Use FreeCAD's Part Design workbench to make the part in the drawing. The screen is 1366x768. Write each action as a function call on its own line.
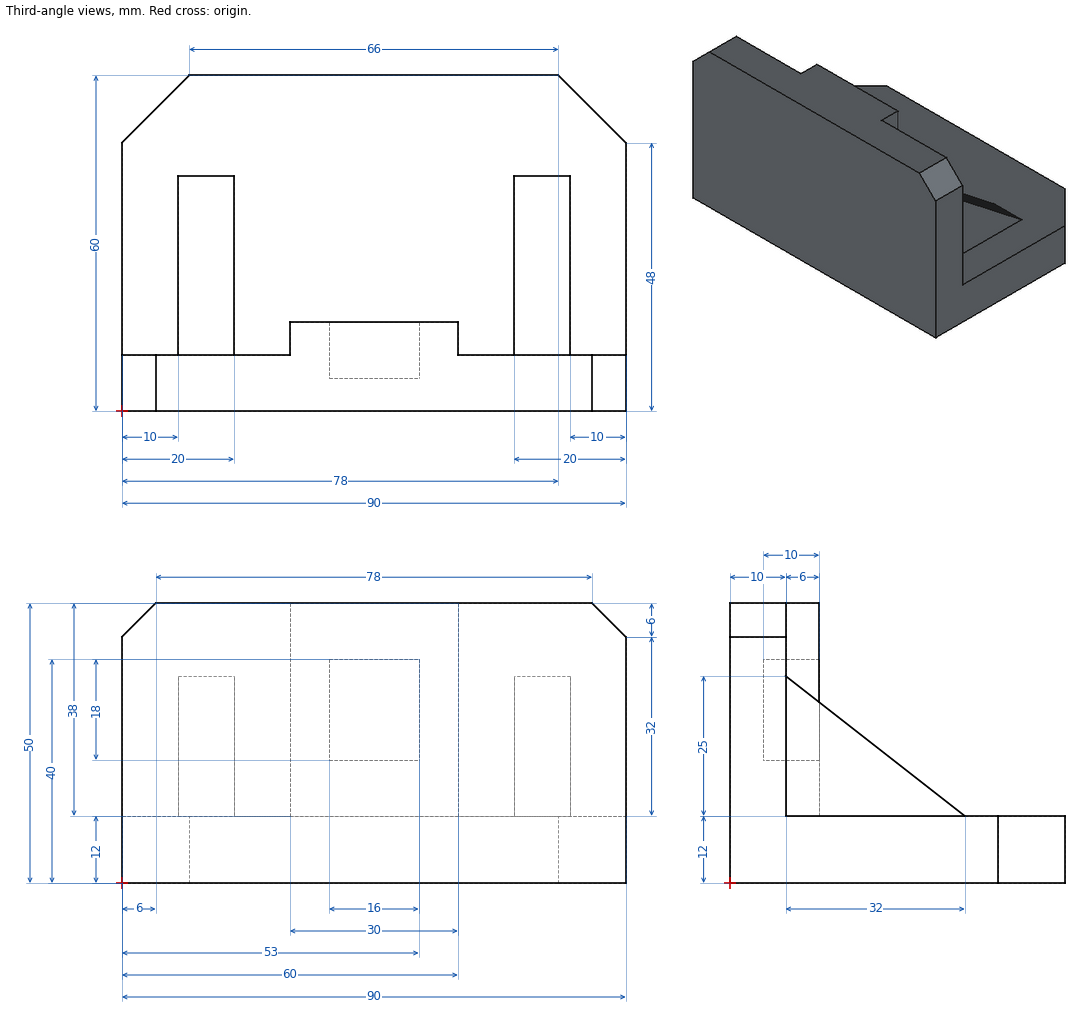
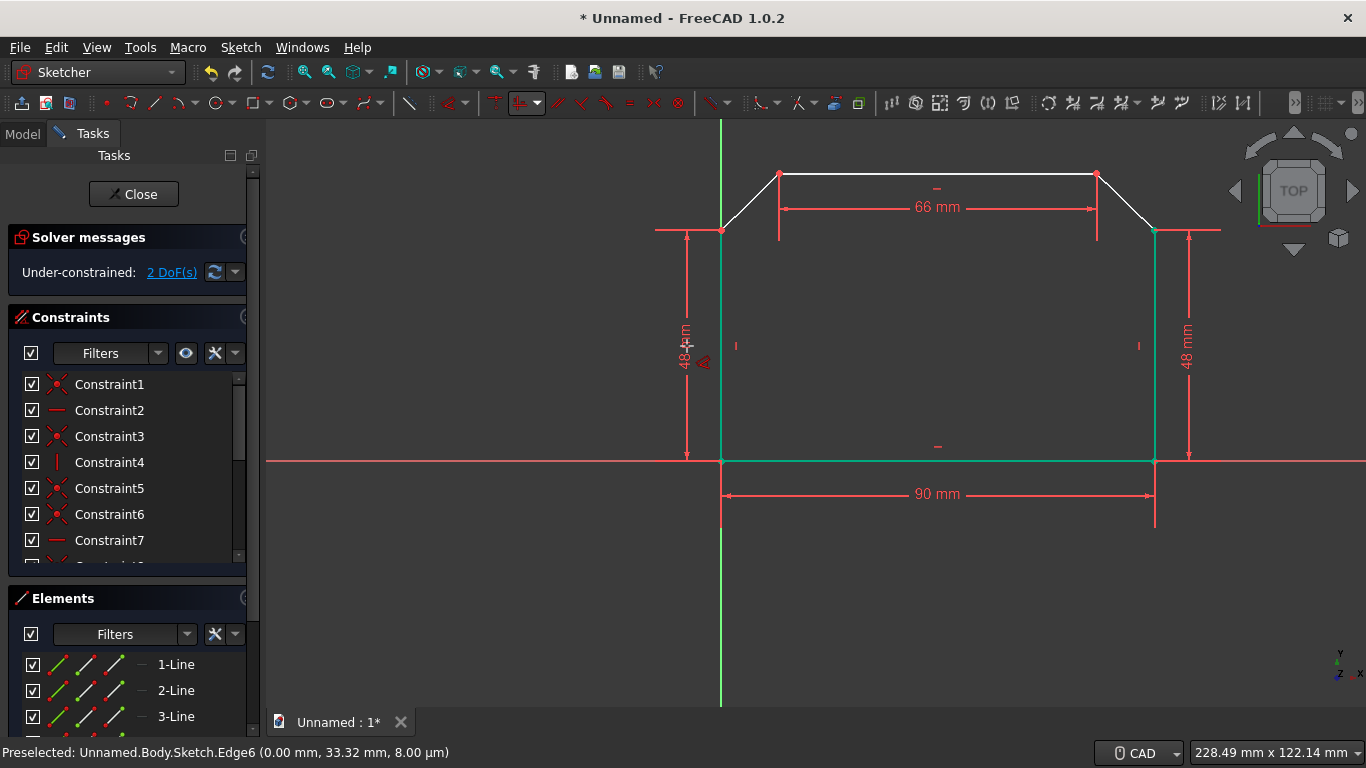
click(1097, 174)
click(823, 495)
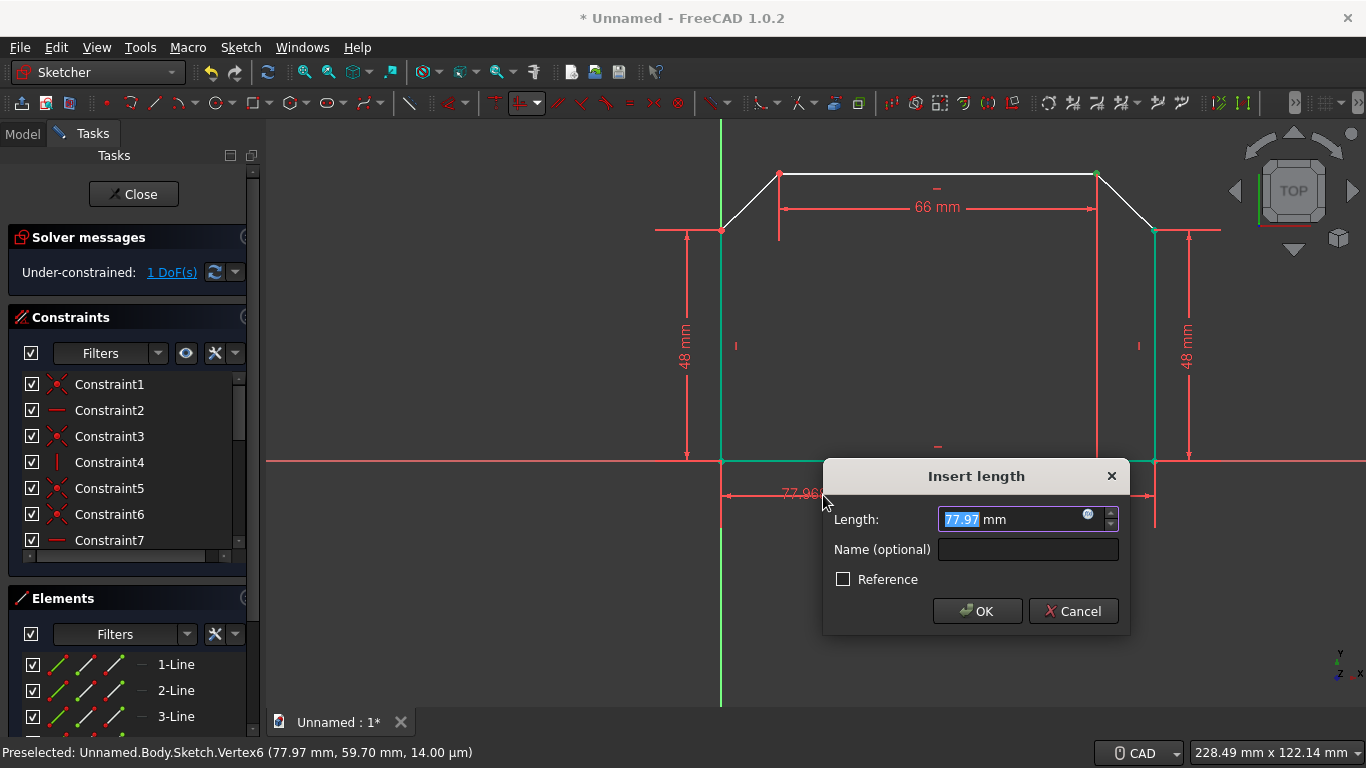
text(78)
key(Return)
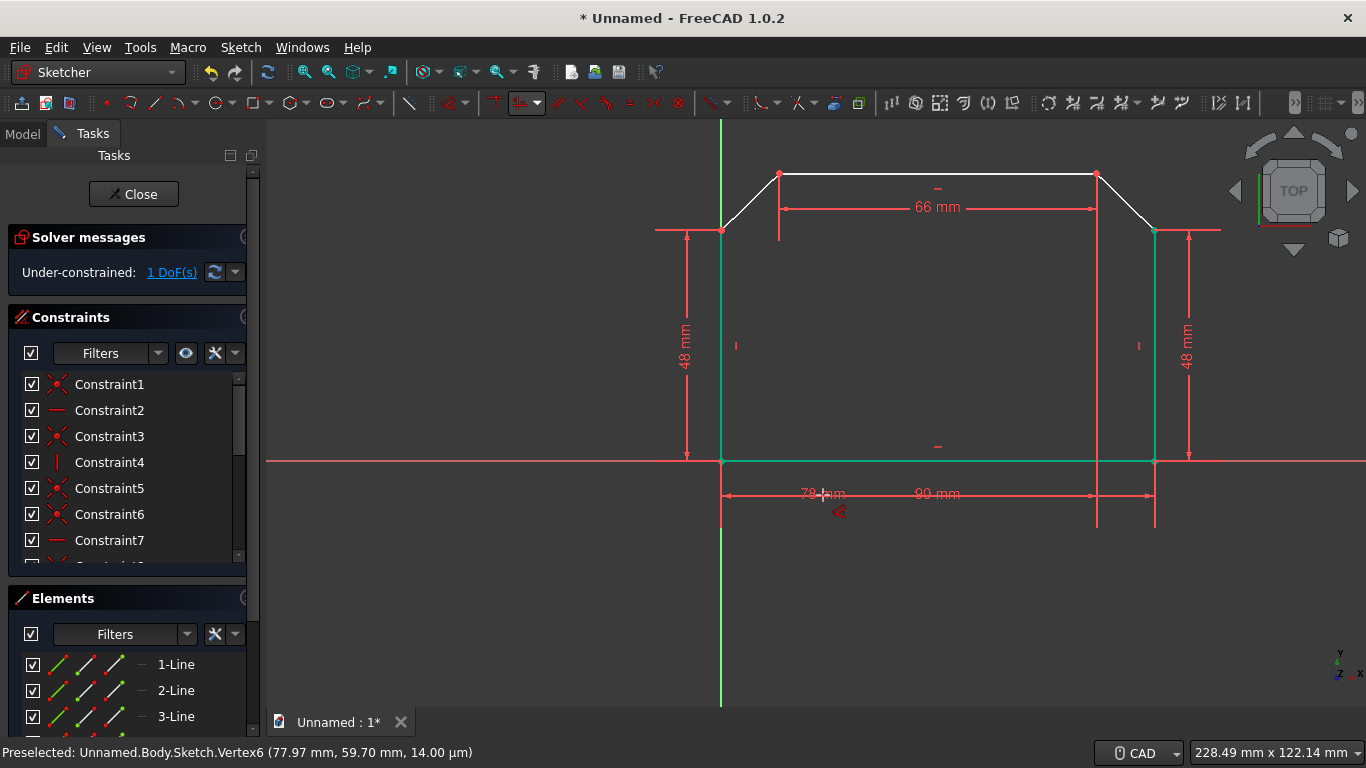
click(1097, 174)
click(687, 318)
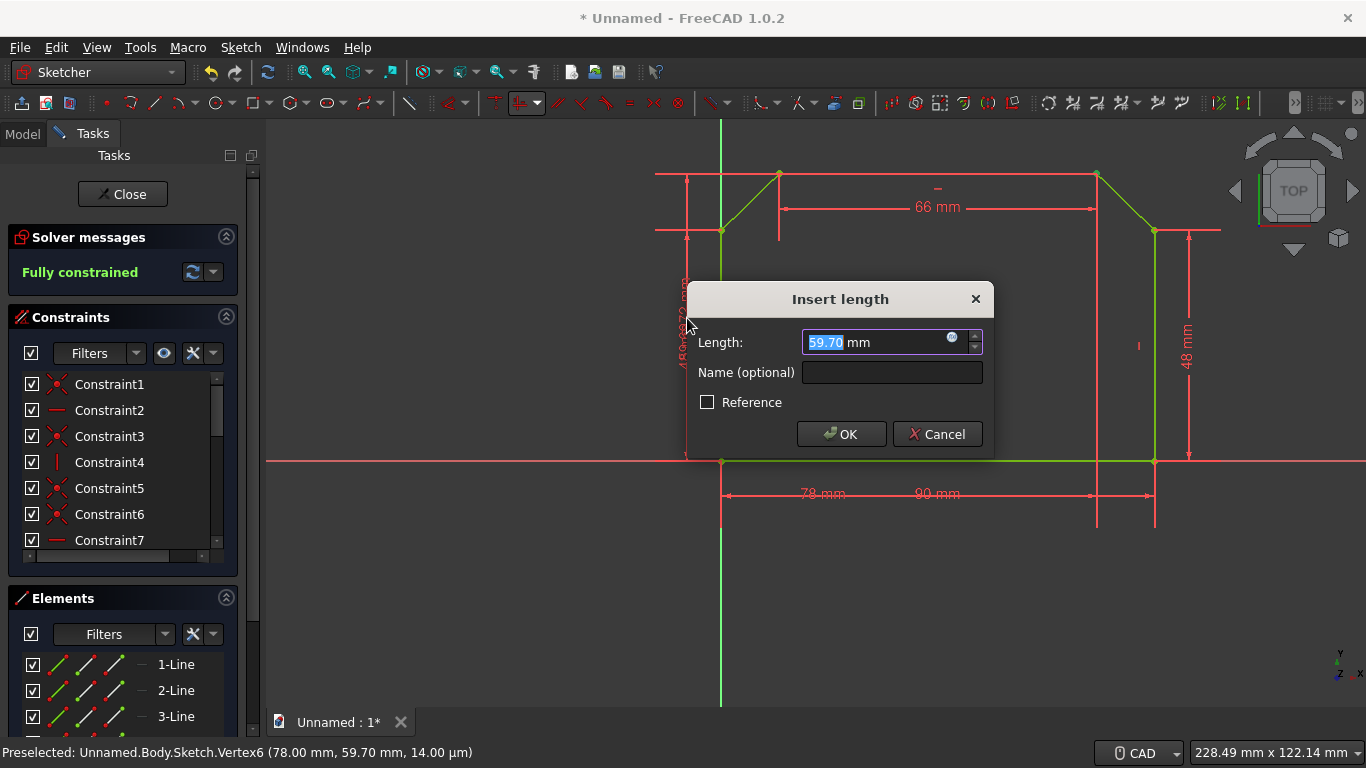
text(60)
key(Return)
key(Escape)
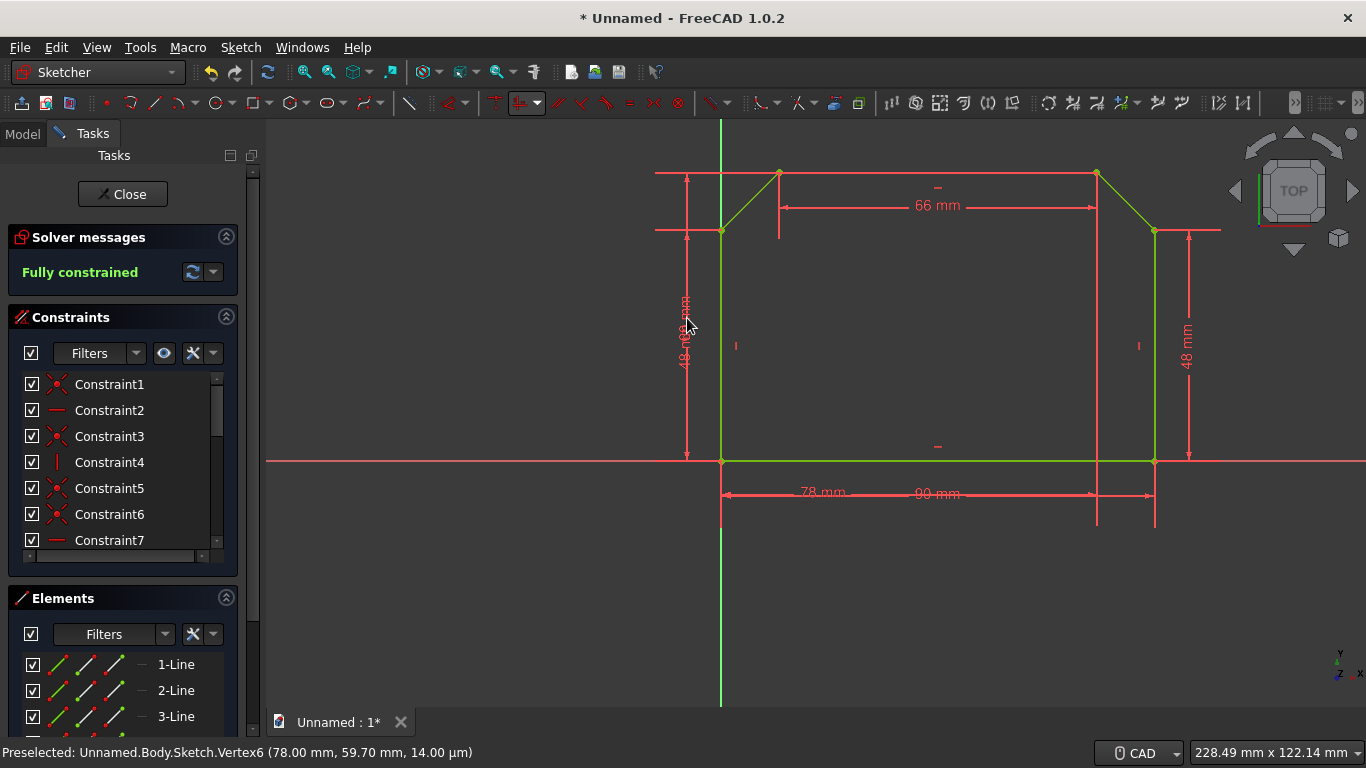
click(123, 194)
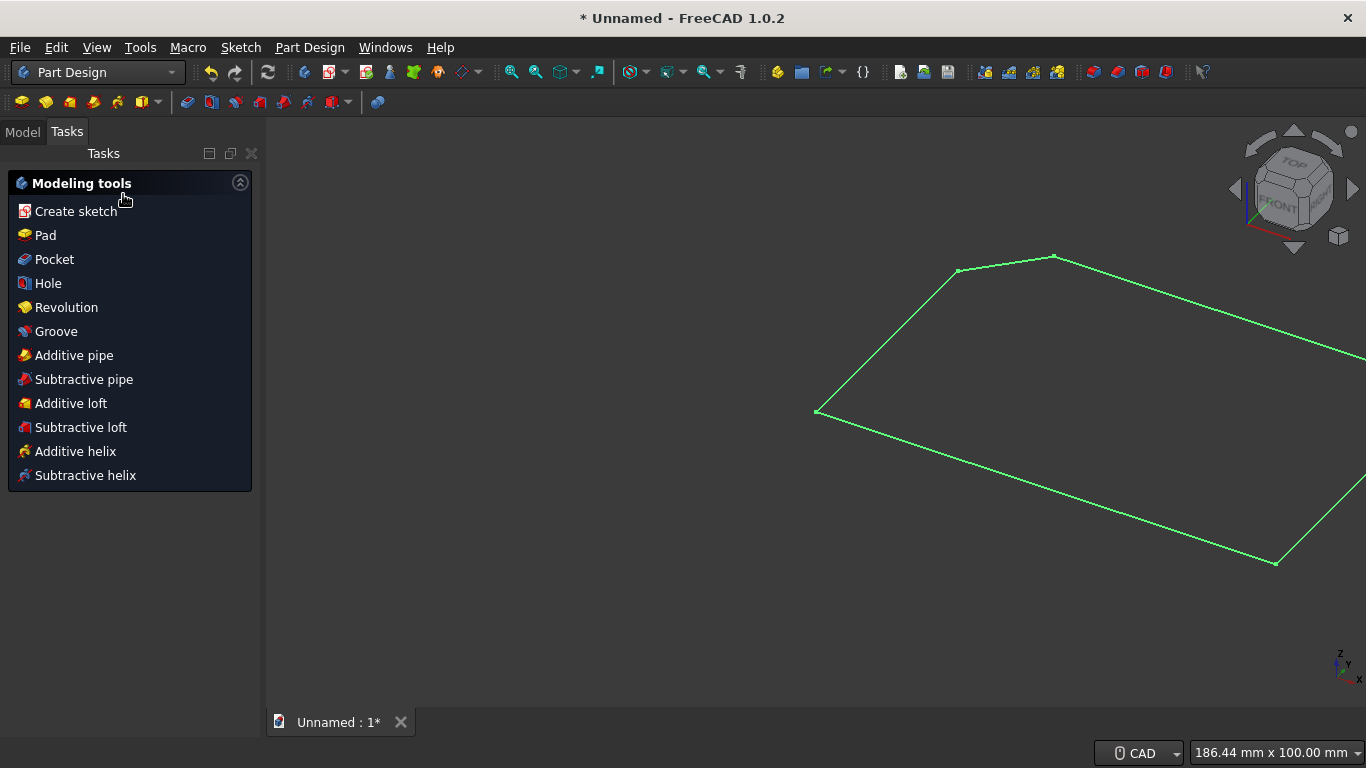
click(22, 102)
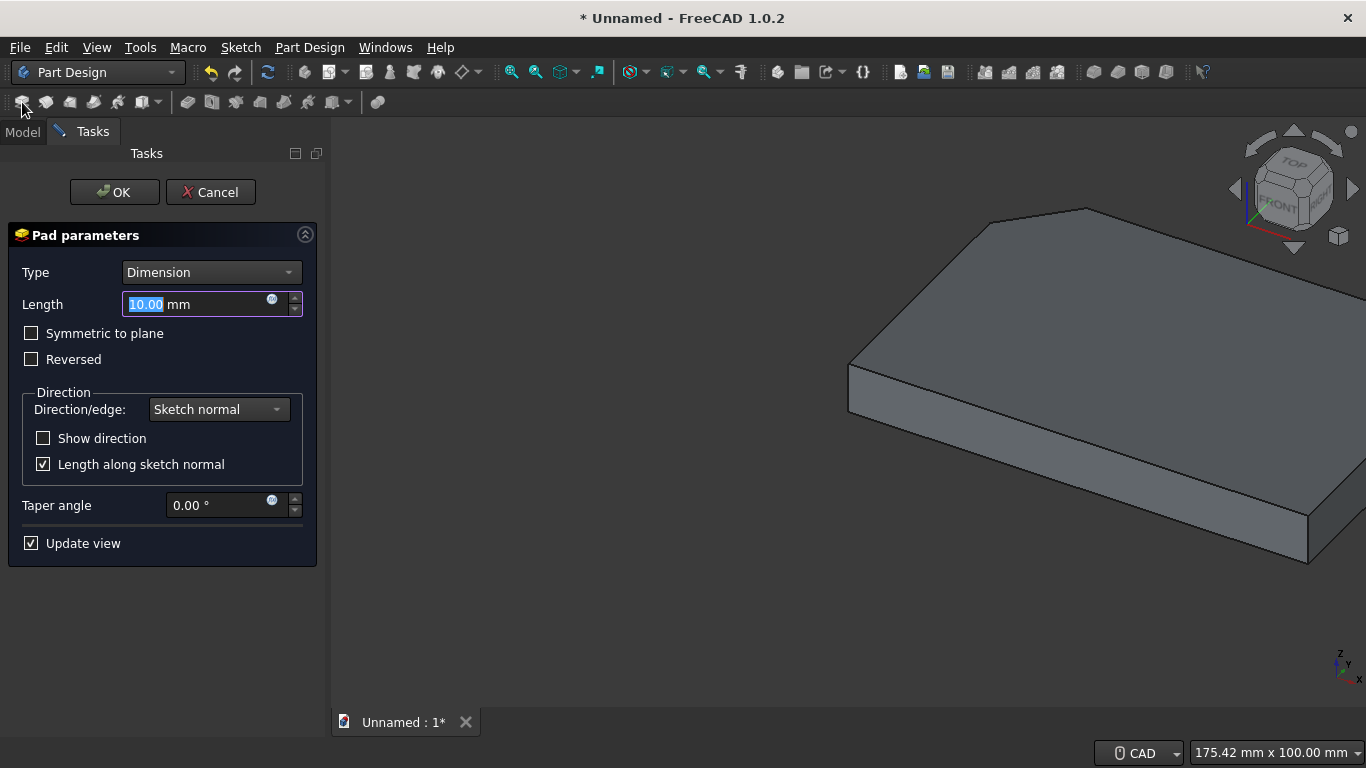
text(12)
key(Tab)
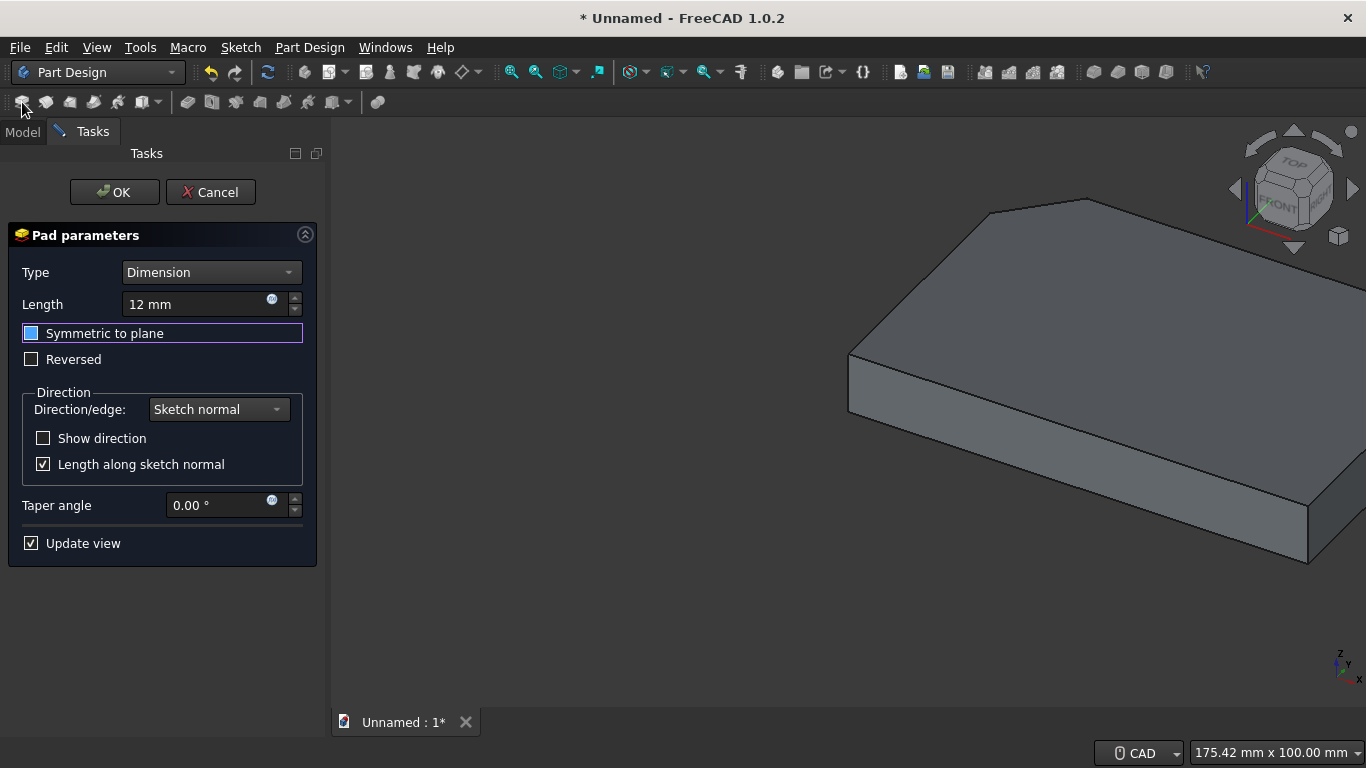
click(115, 192)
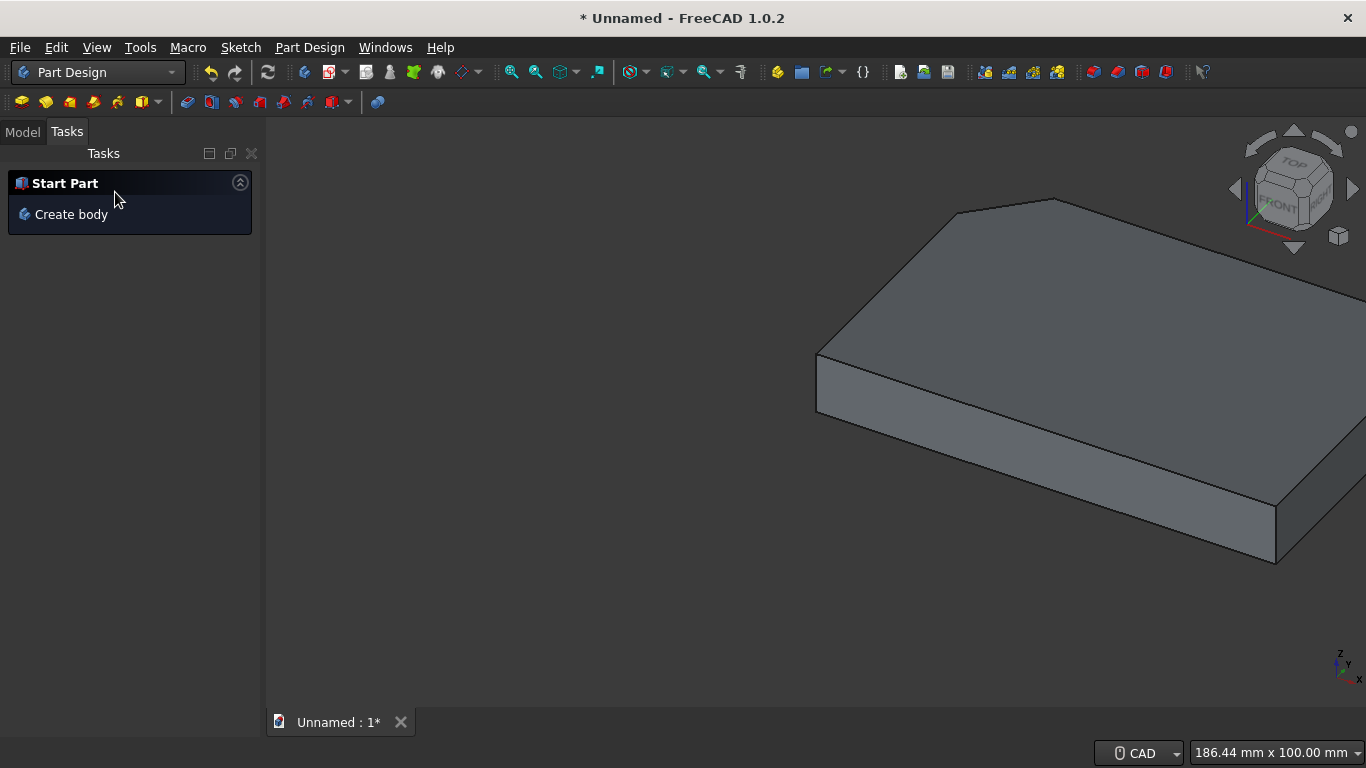
click(512, 72)